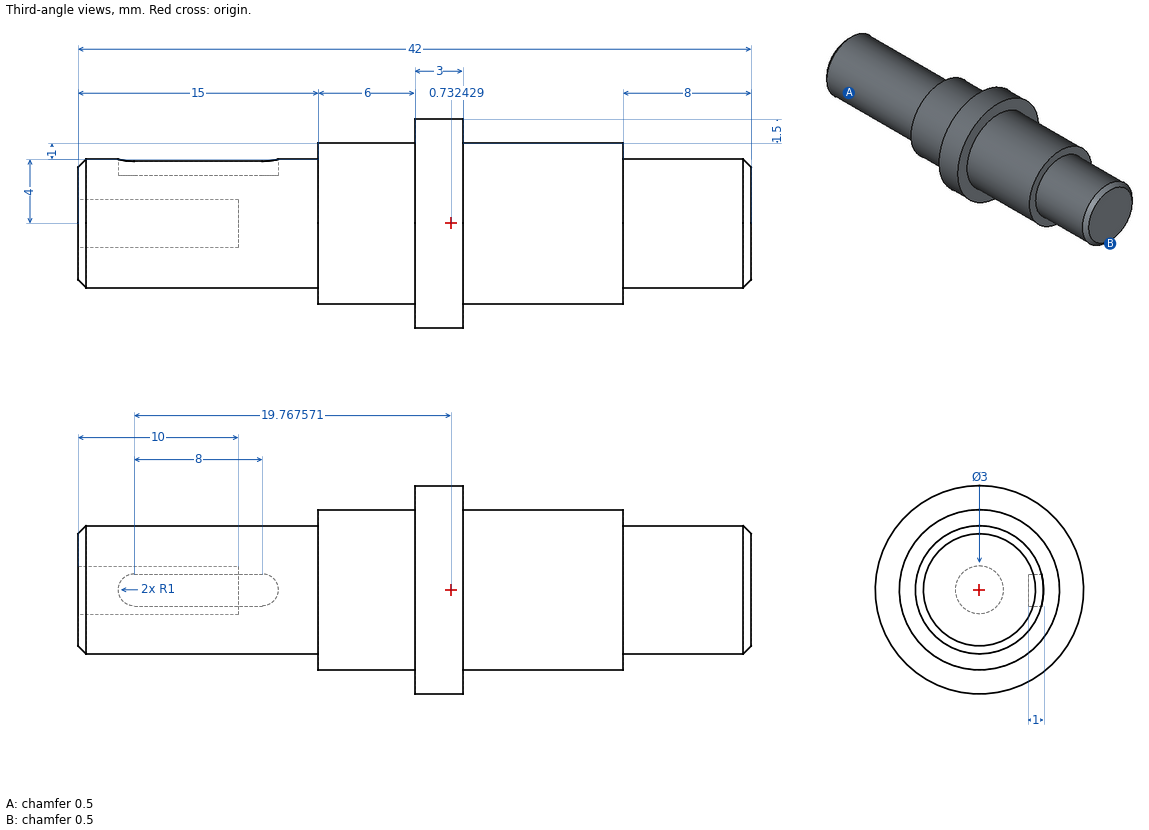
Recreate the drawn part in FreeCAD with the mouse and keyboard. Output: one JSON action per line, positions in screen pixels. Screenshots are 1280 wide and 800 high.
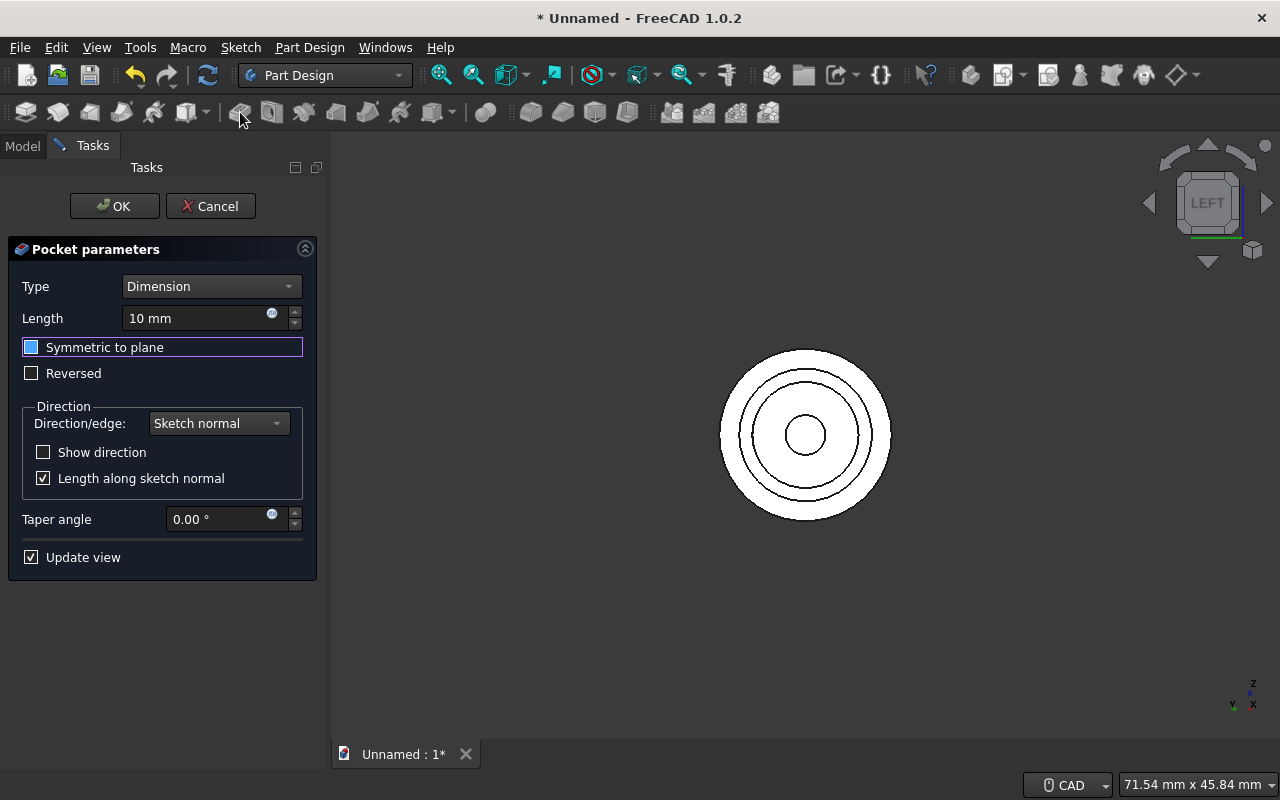
{"action": "left_click", "coordinate": [115, 206]}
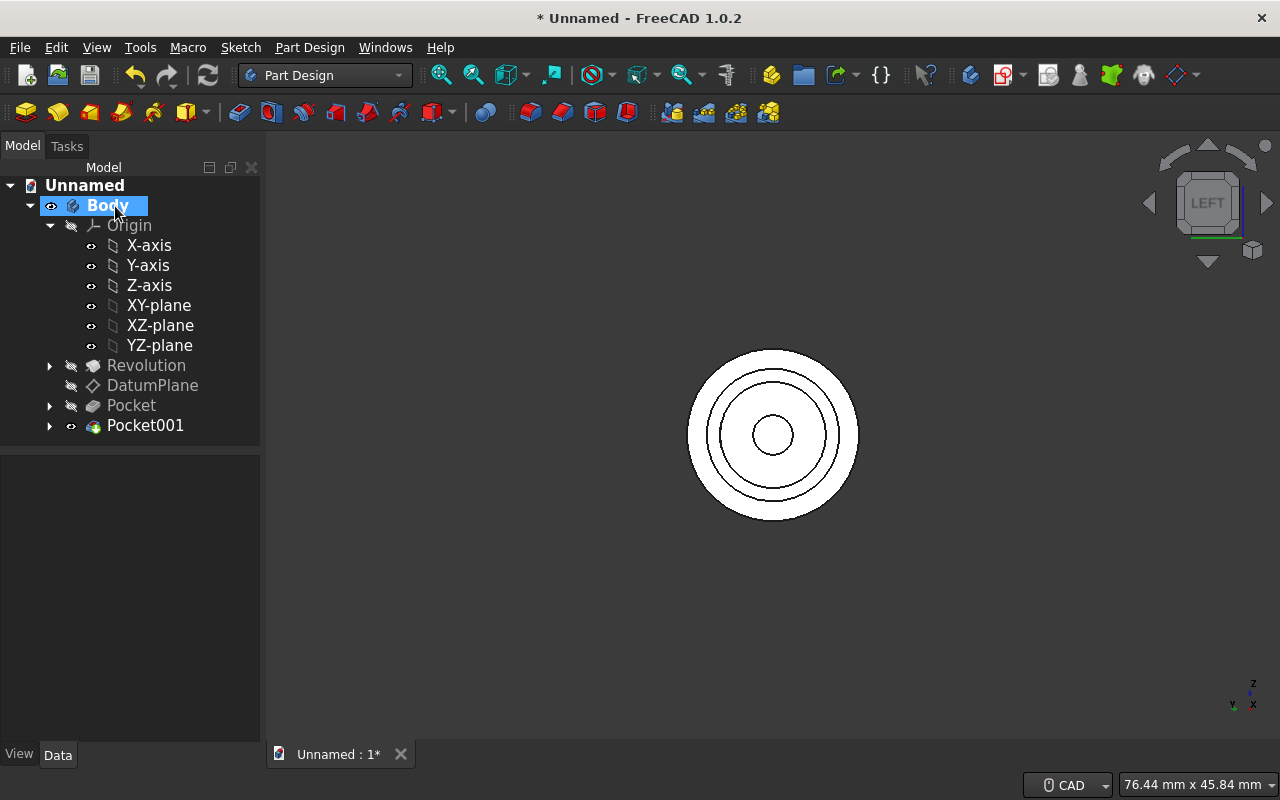
{"action": "left_click", "coordinate": [442, 76]}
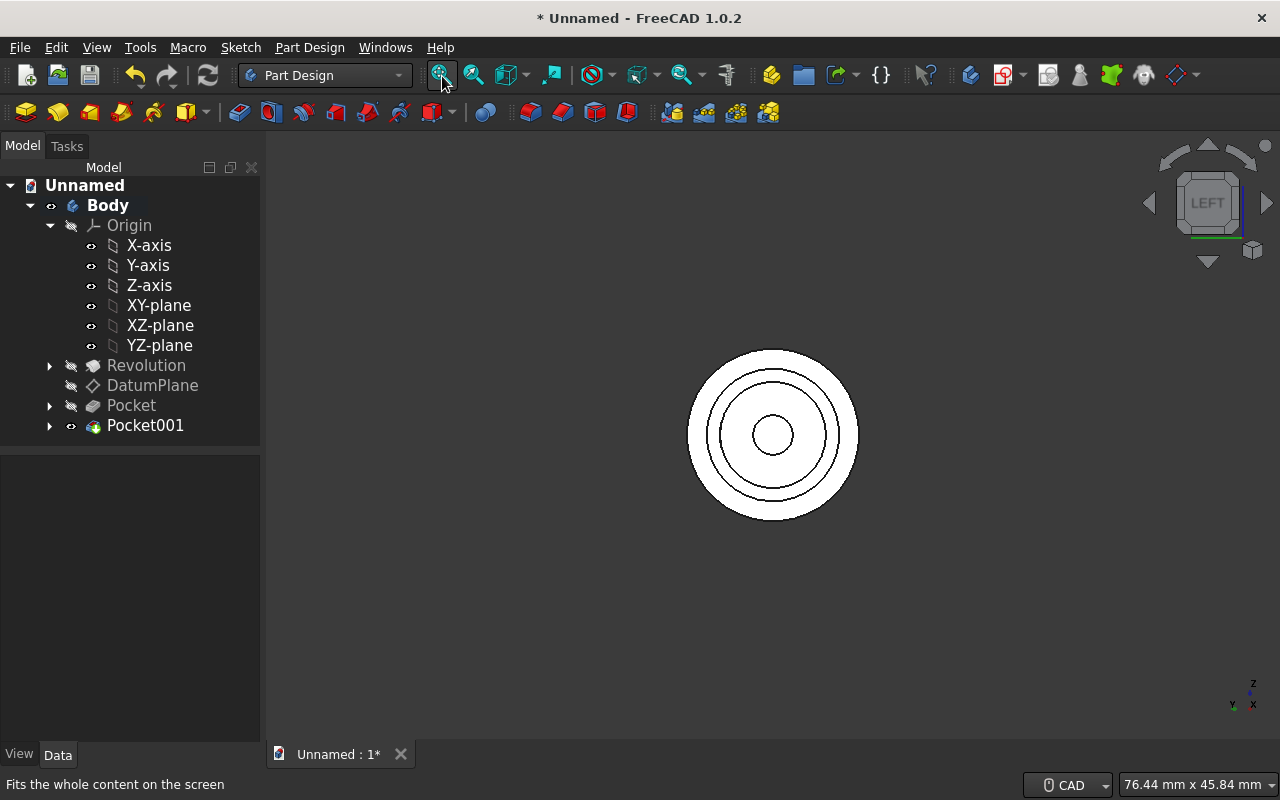
{"action": "left_click", "coordinate": [826, 434]}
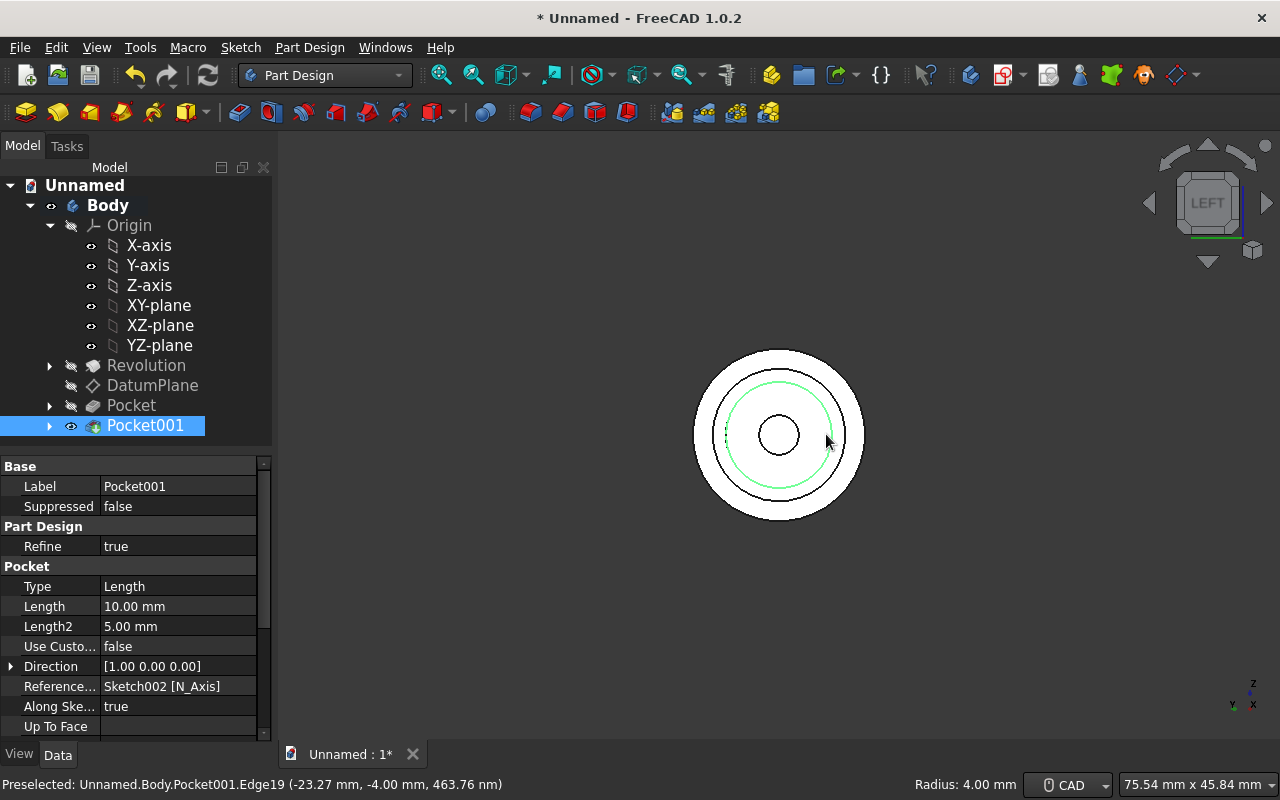
{"action": "left_click", "coordinate": [564, 112]}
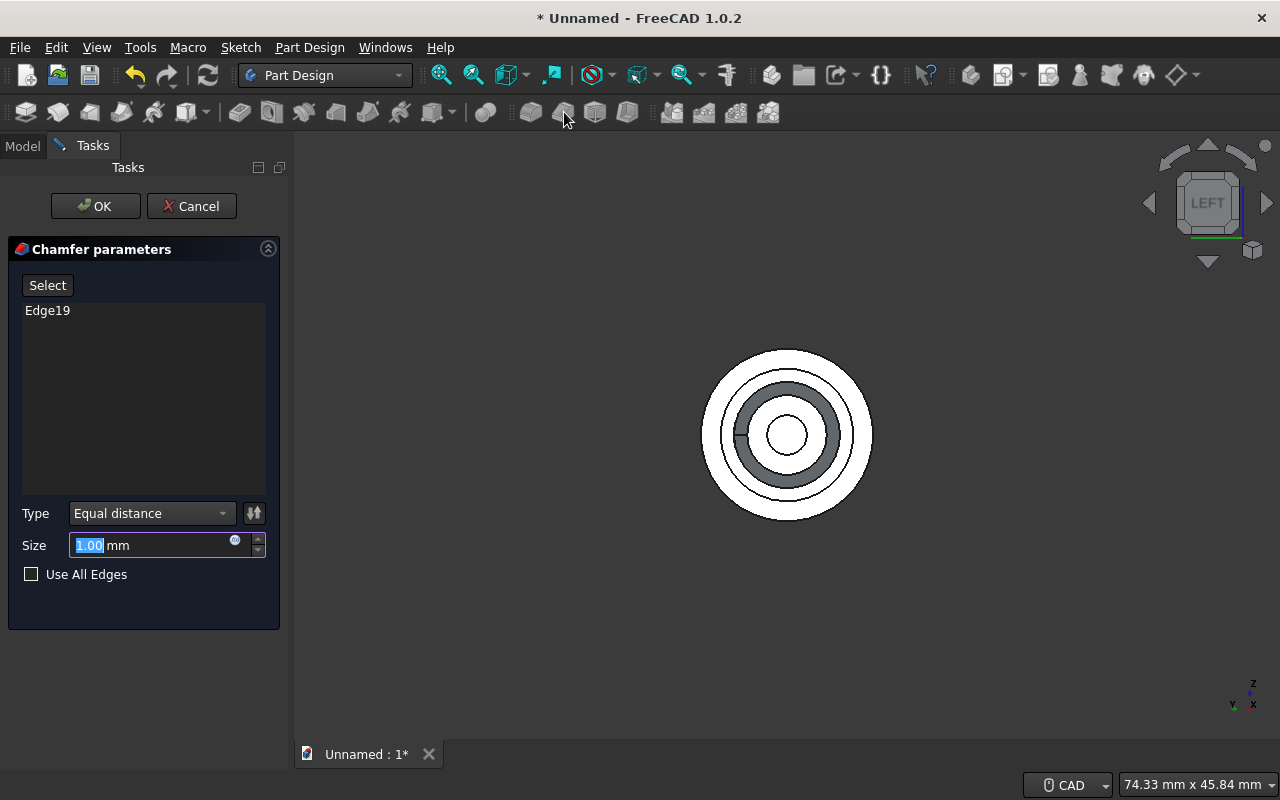
{"action": "type", "text": "0.5"}
{"action": "key", "text": "Tab"}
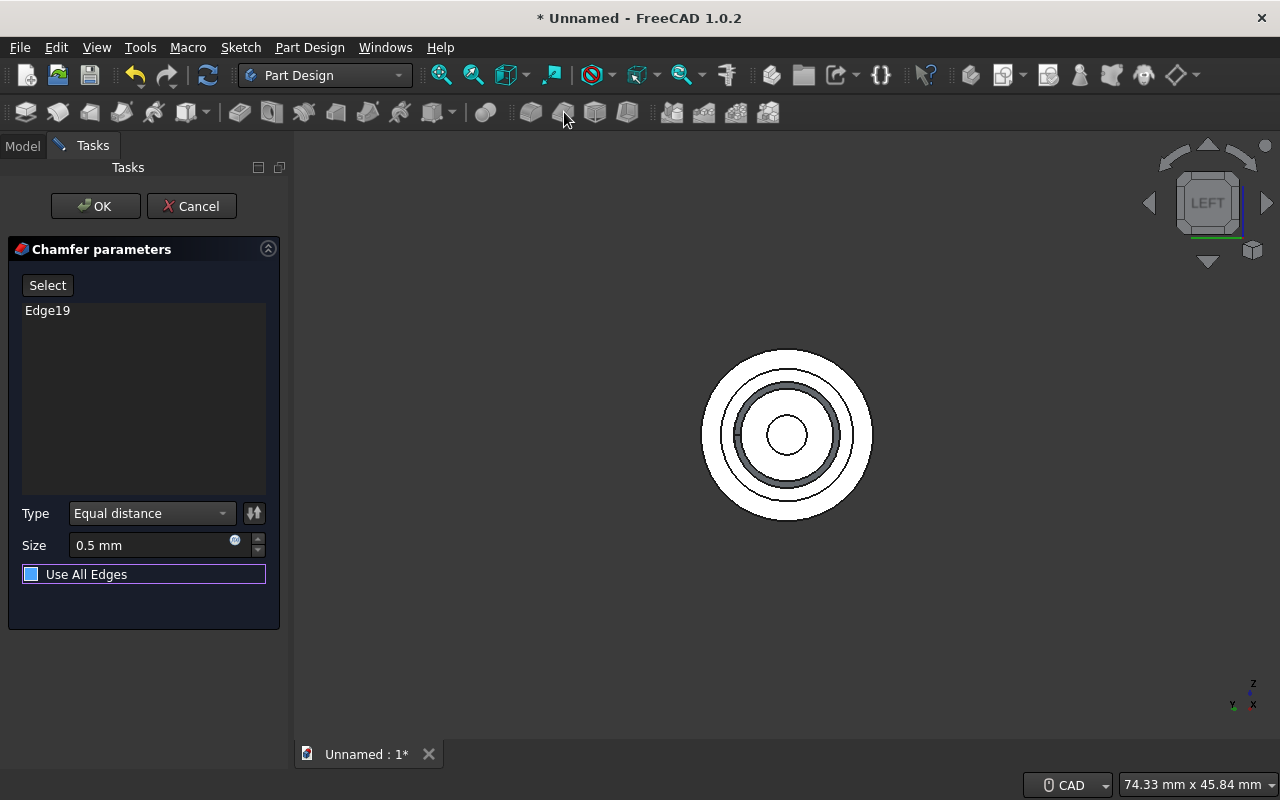
{"action": "left_click", "coordinate": [96, 206]}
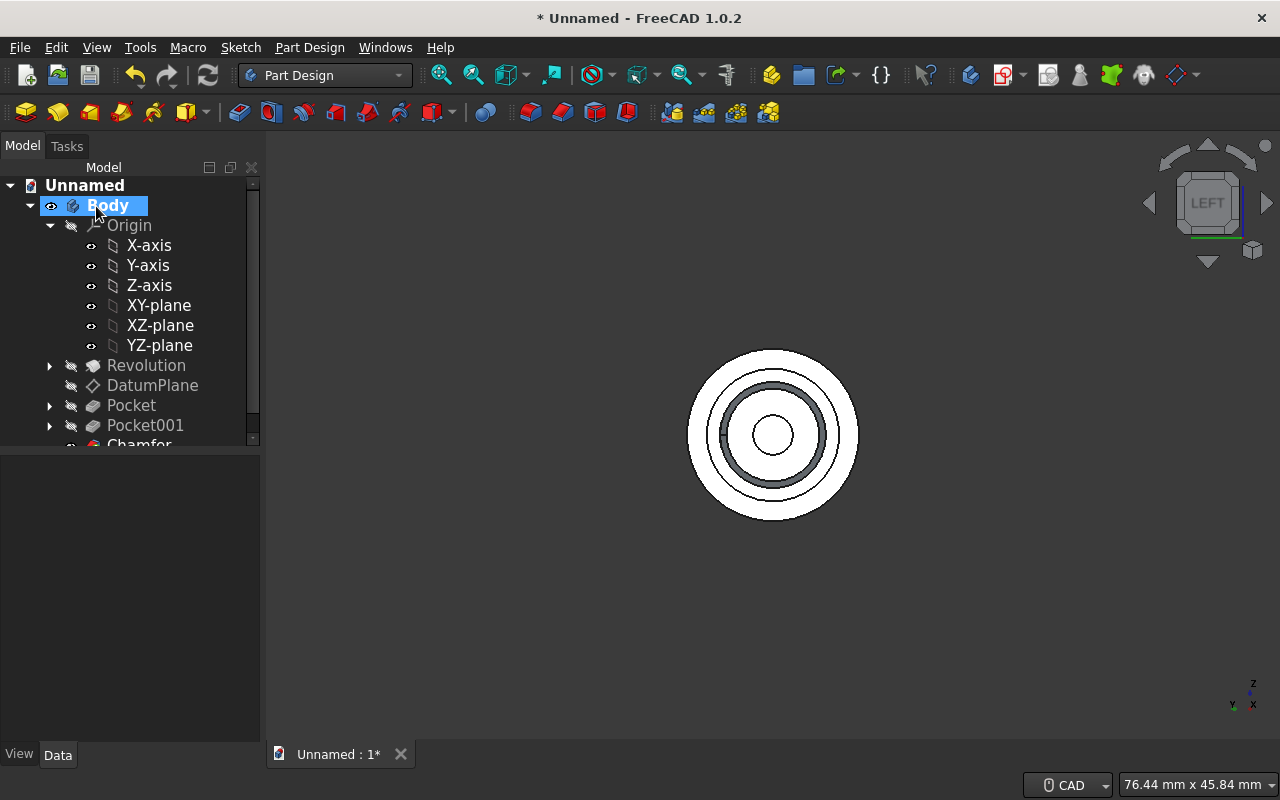
{"action": "left_click", "coordinate": [442, 76]}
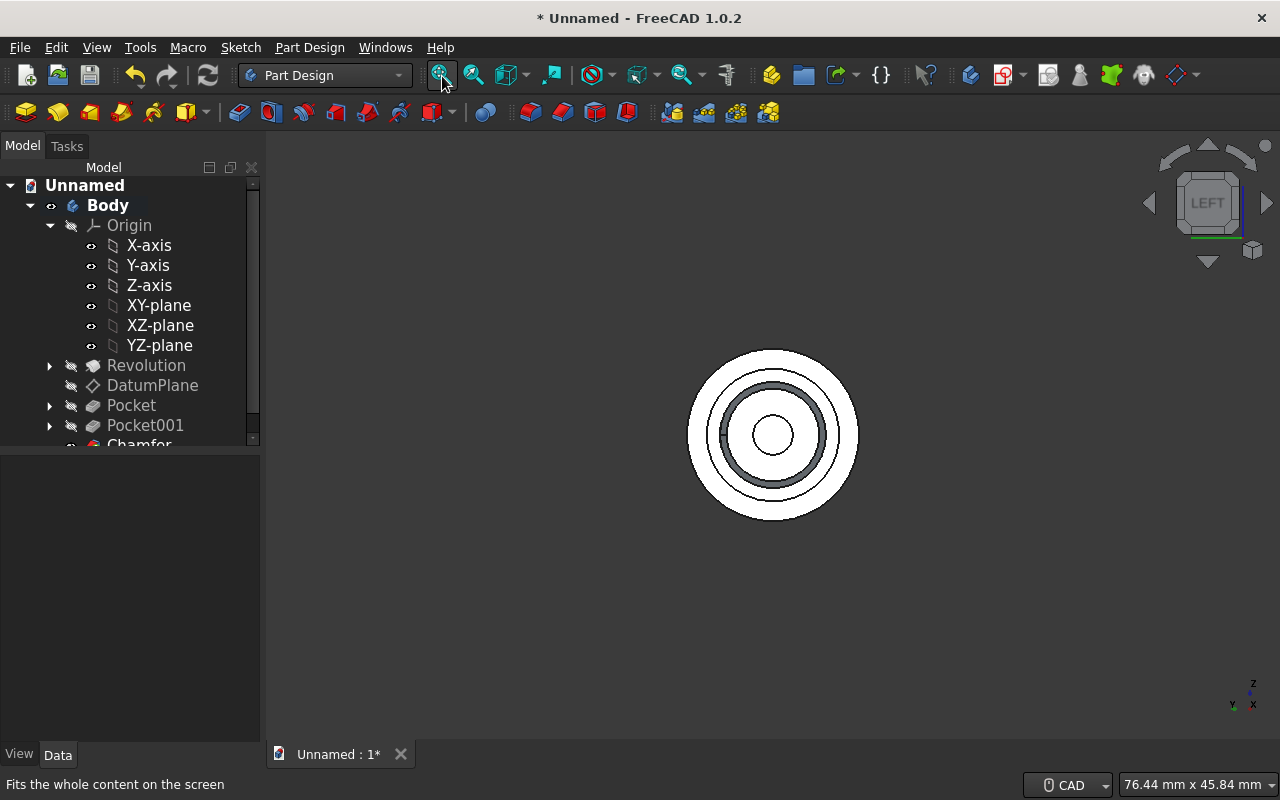
{"action": "key", "text": "0"}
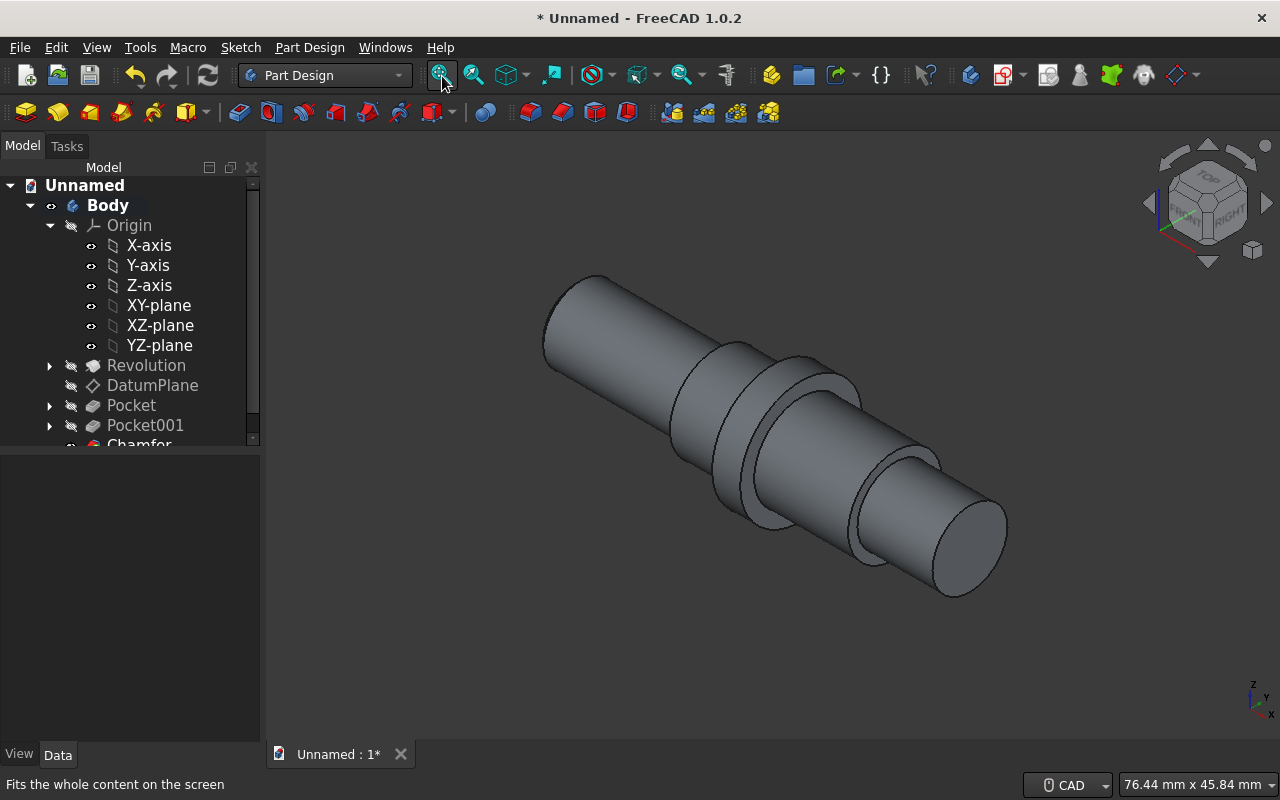
{"action": "left_click", "coordinate": [932, 569]}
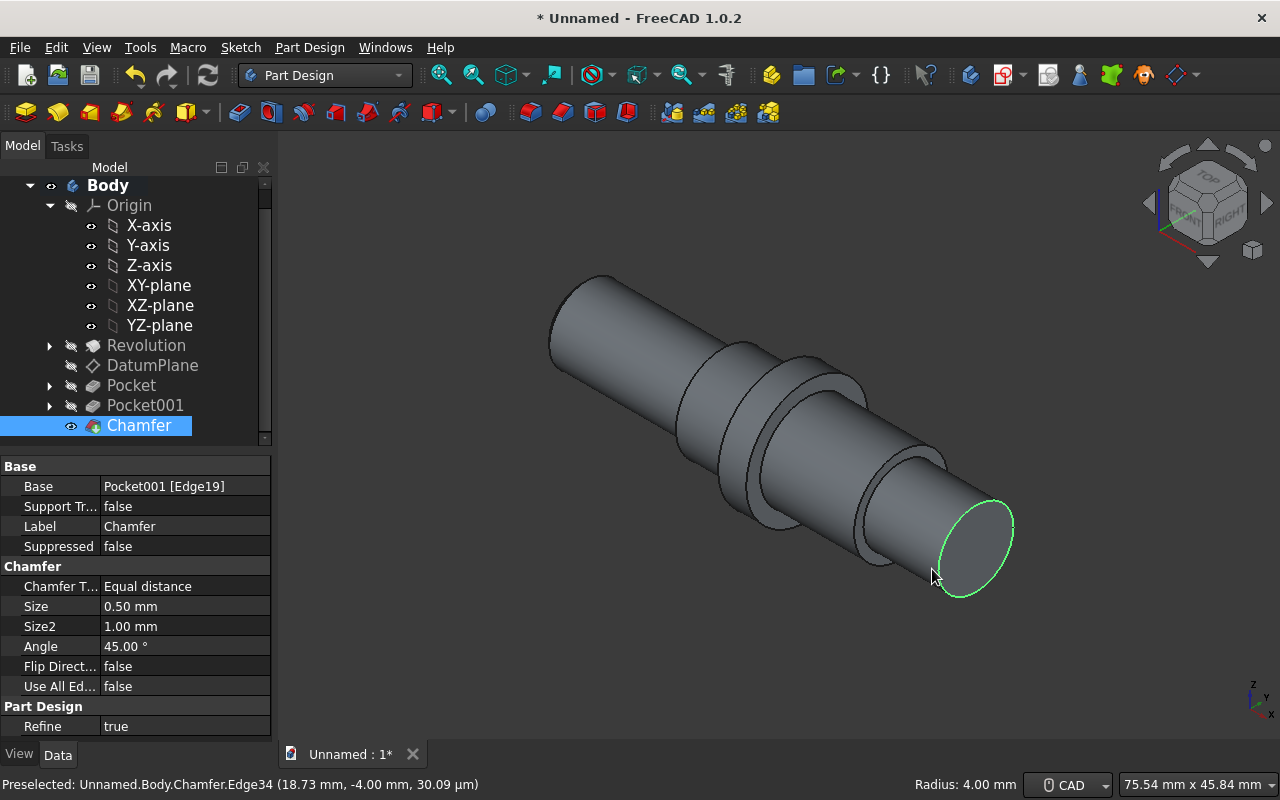
{"action": "left_click", "coordinate": [564, 112]}